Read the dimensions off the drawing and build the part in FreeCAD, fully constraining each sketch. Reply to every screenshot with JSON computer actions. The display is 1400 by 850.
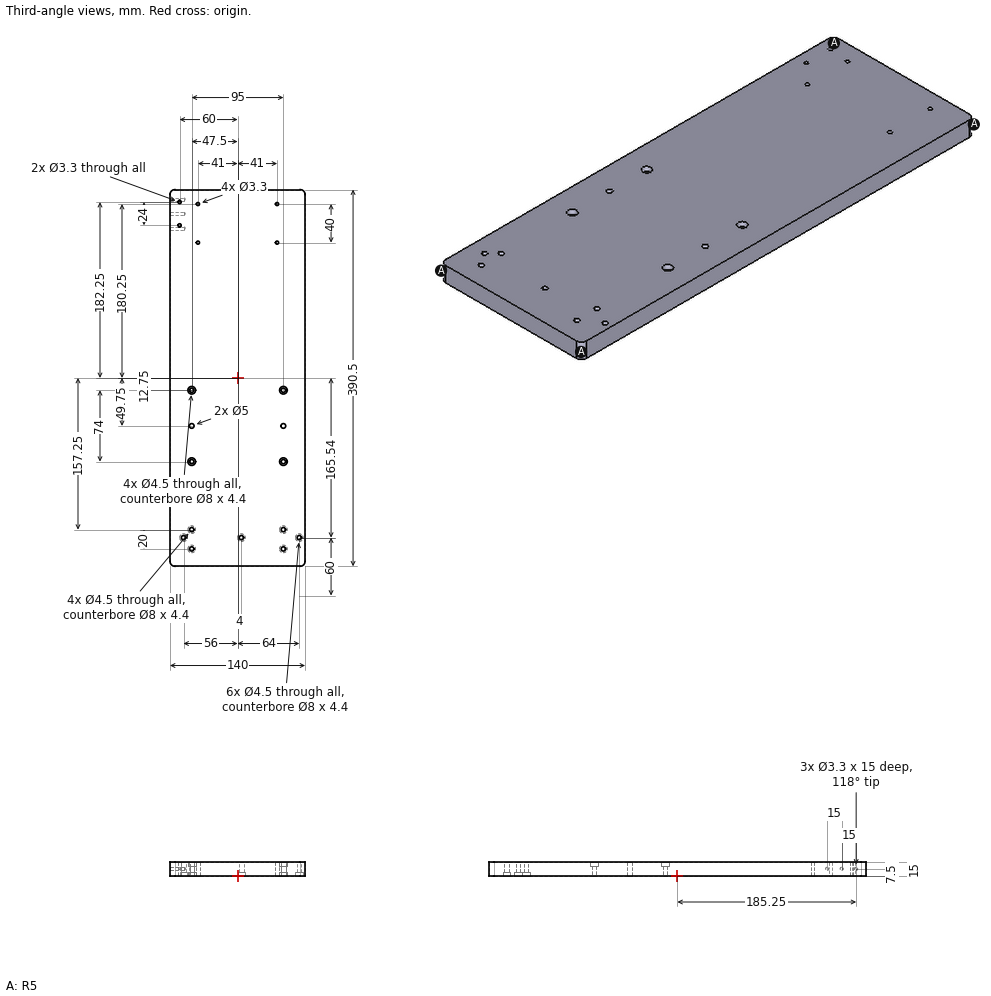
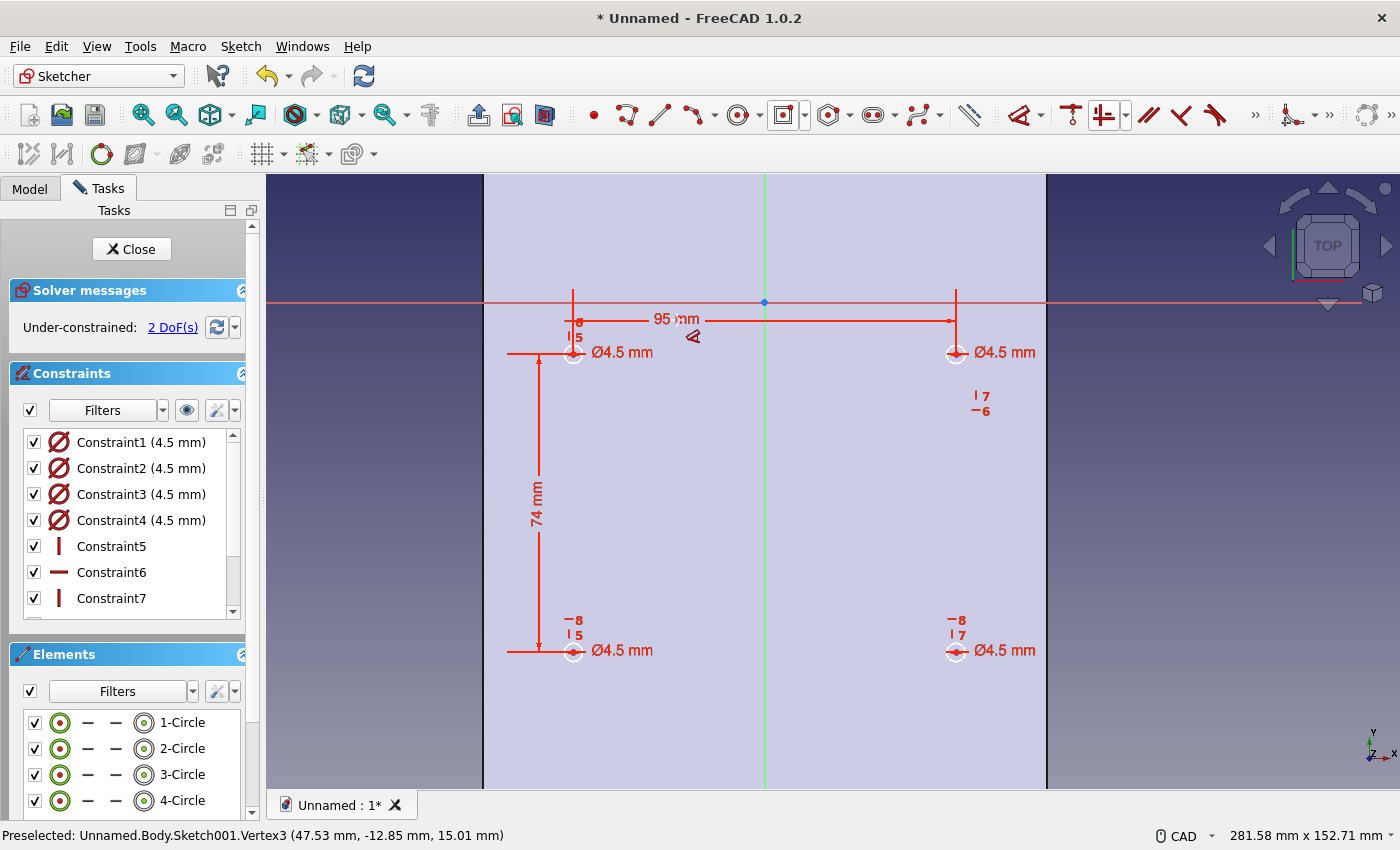
{"action": "left_click", "coordinate": [573, 354]}
{"action": "left_click", "coordinate": [669, 269]}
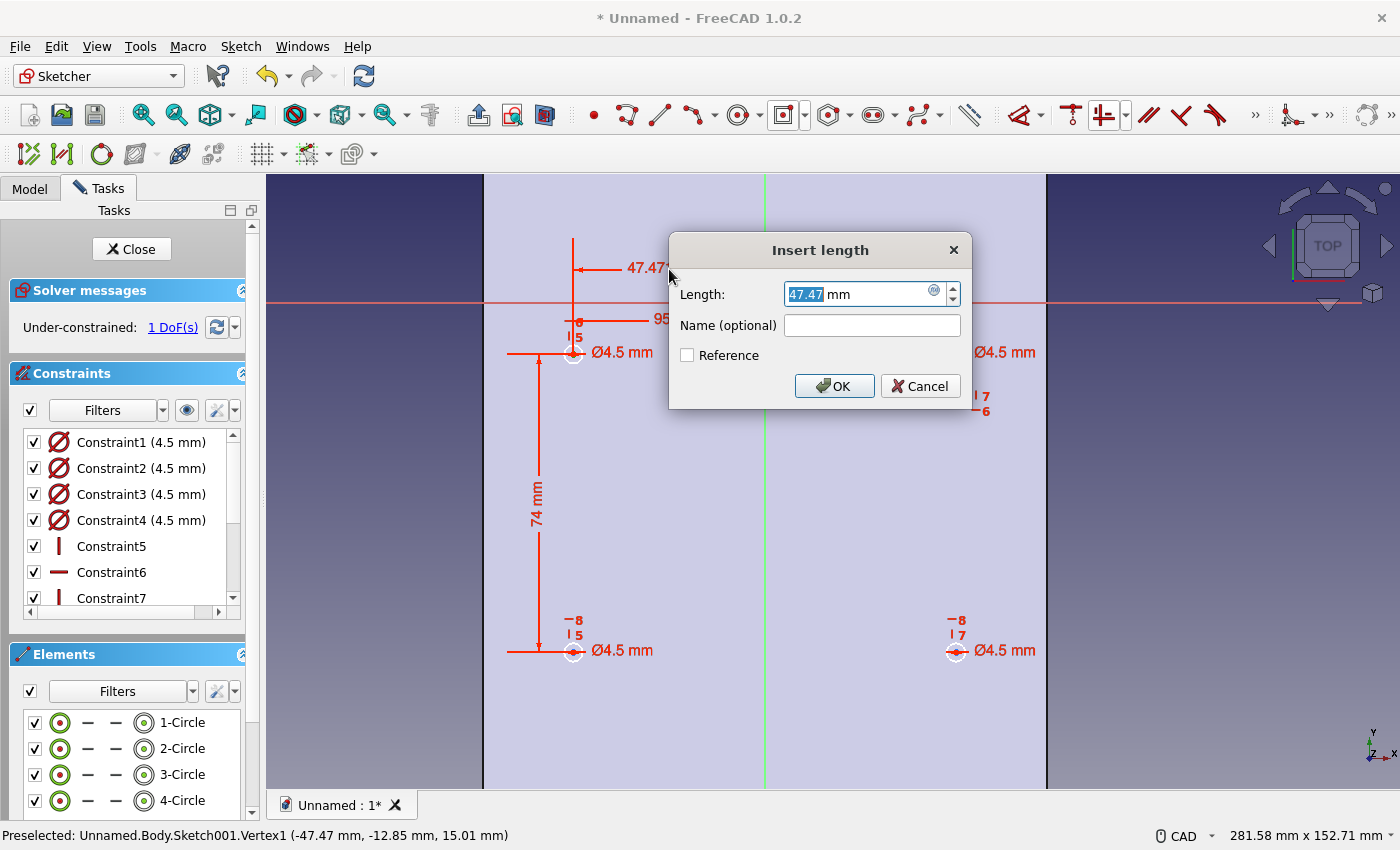
{"action": "type", "text": "47.5"}
{"action": "key", "text": "Return"}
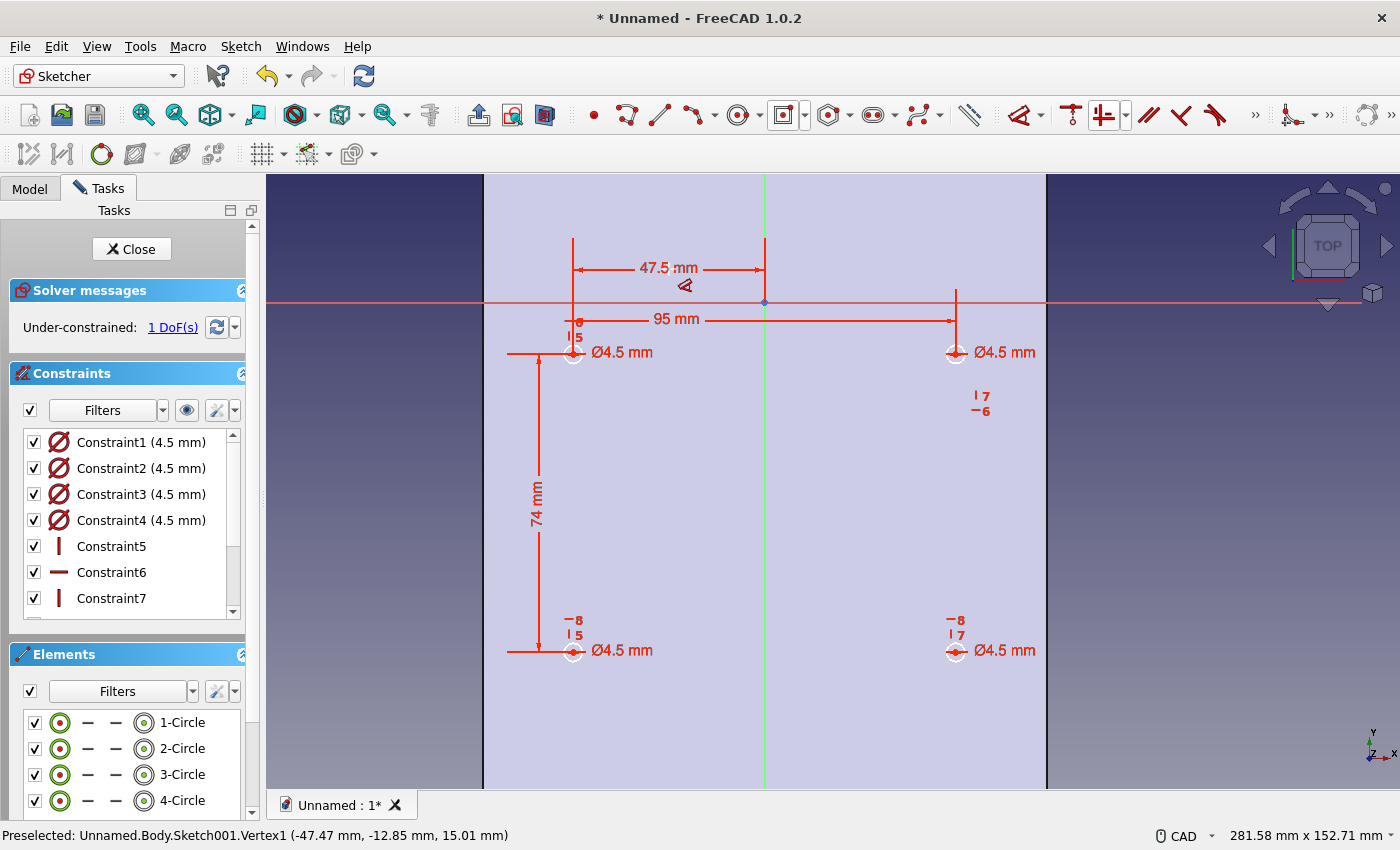
{"action": "left_click", "coordinate": [573, 354]}
{"action": "left_click", "coordinate": [539, 329]}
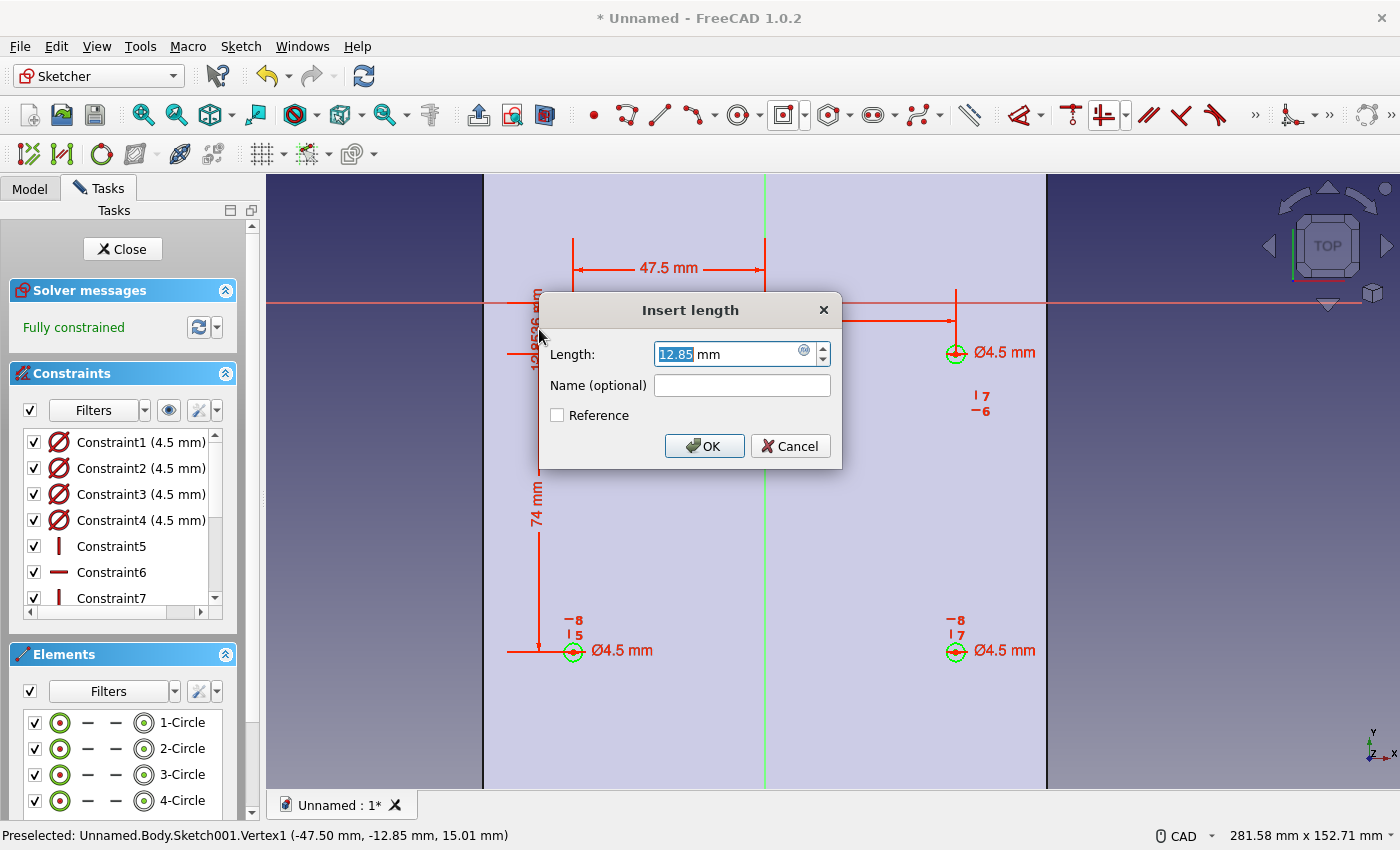
{"action": "type", "text": "12.75"}
{"action": "key", "text": "Return"}
{"action": "key", "text": "Escape"}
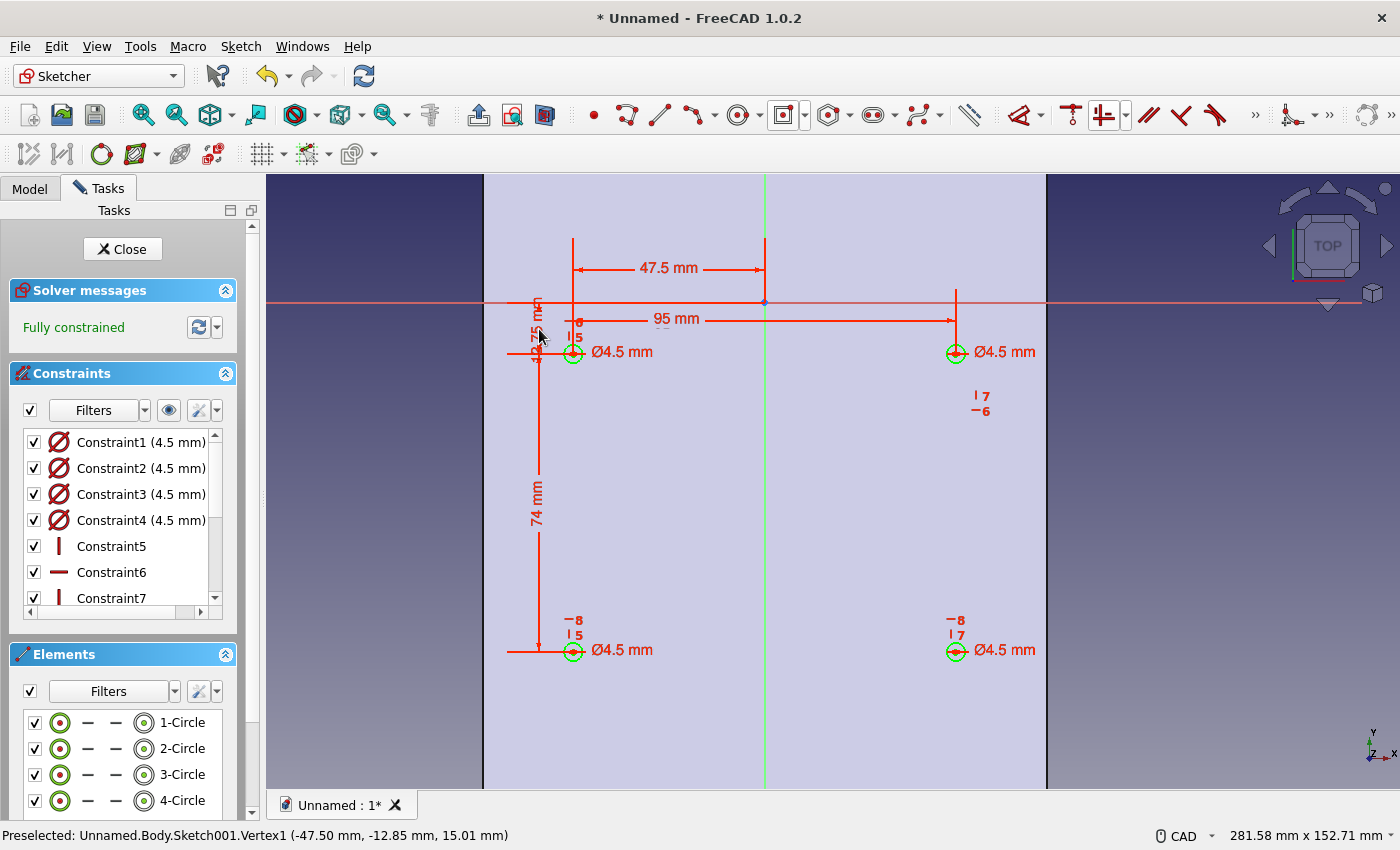
{"action": "left_click", "coordinate": [123, 249]}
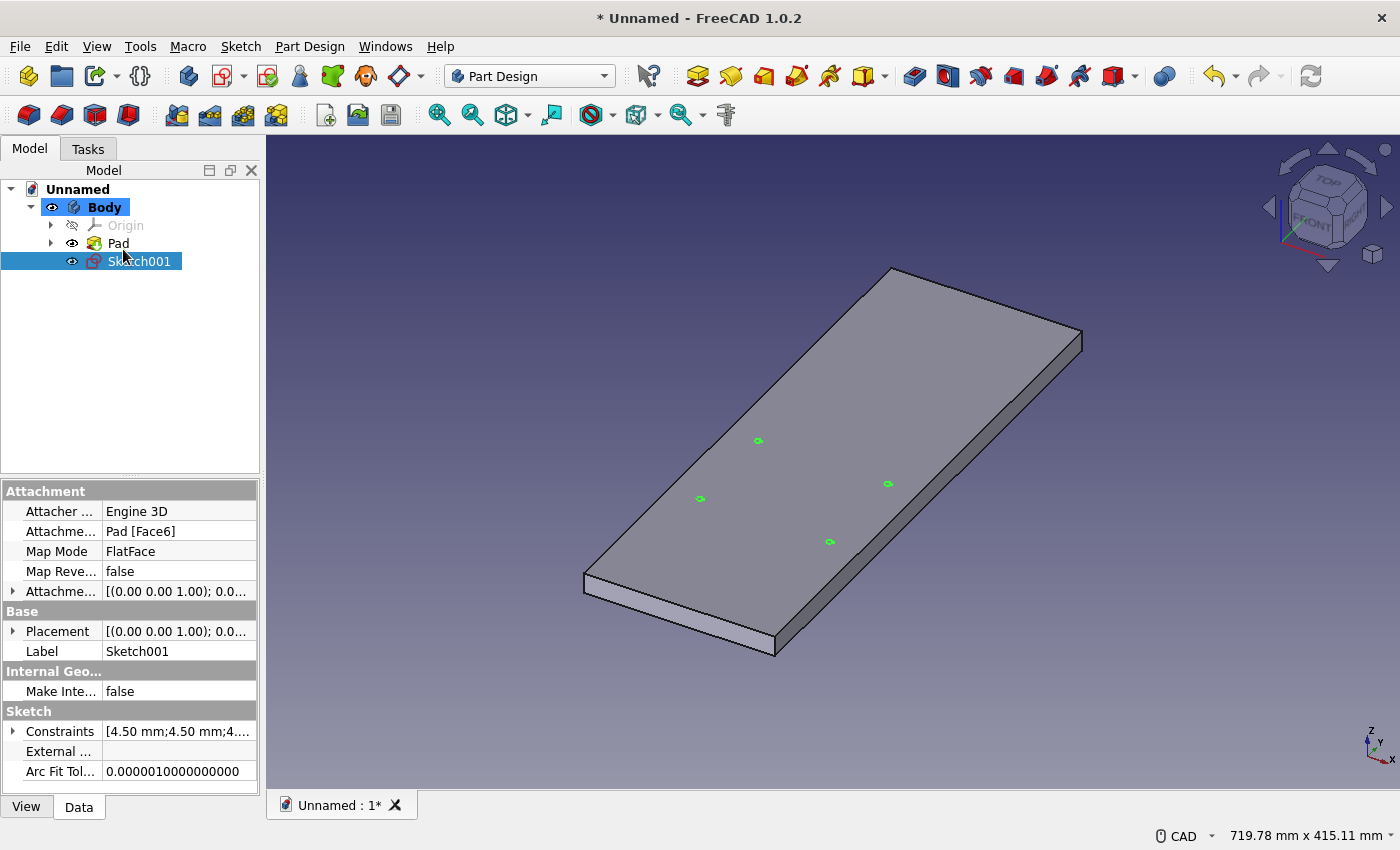
{"action": "left_click", "coordinate": [948, 76]}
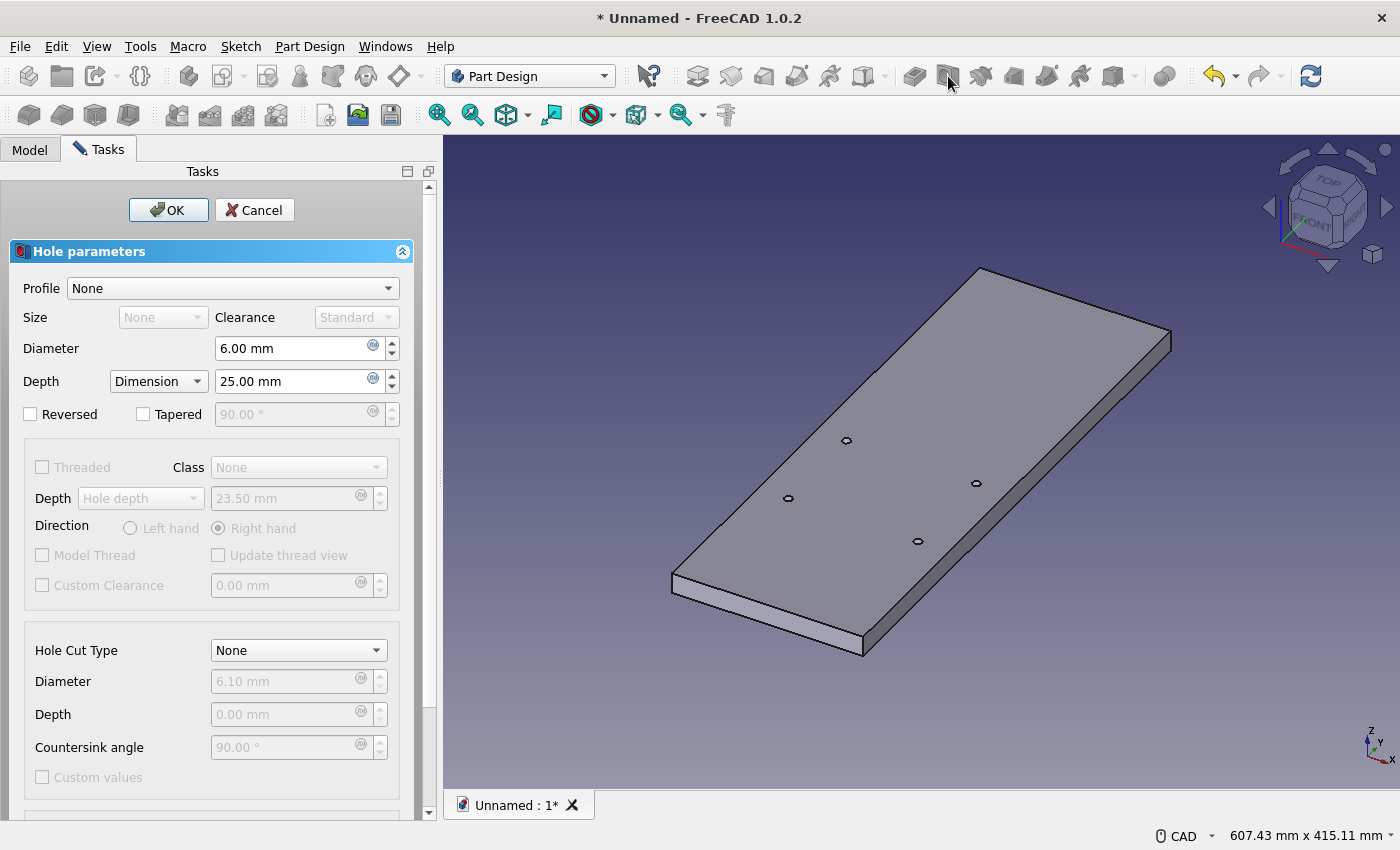
{"action": "triple_click", "coordinate": [300, 348]}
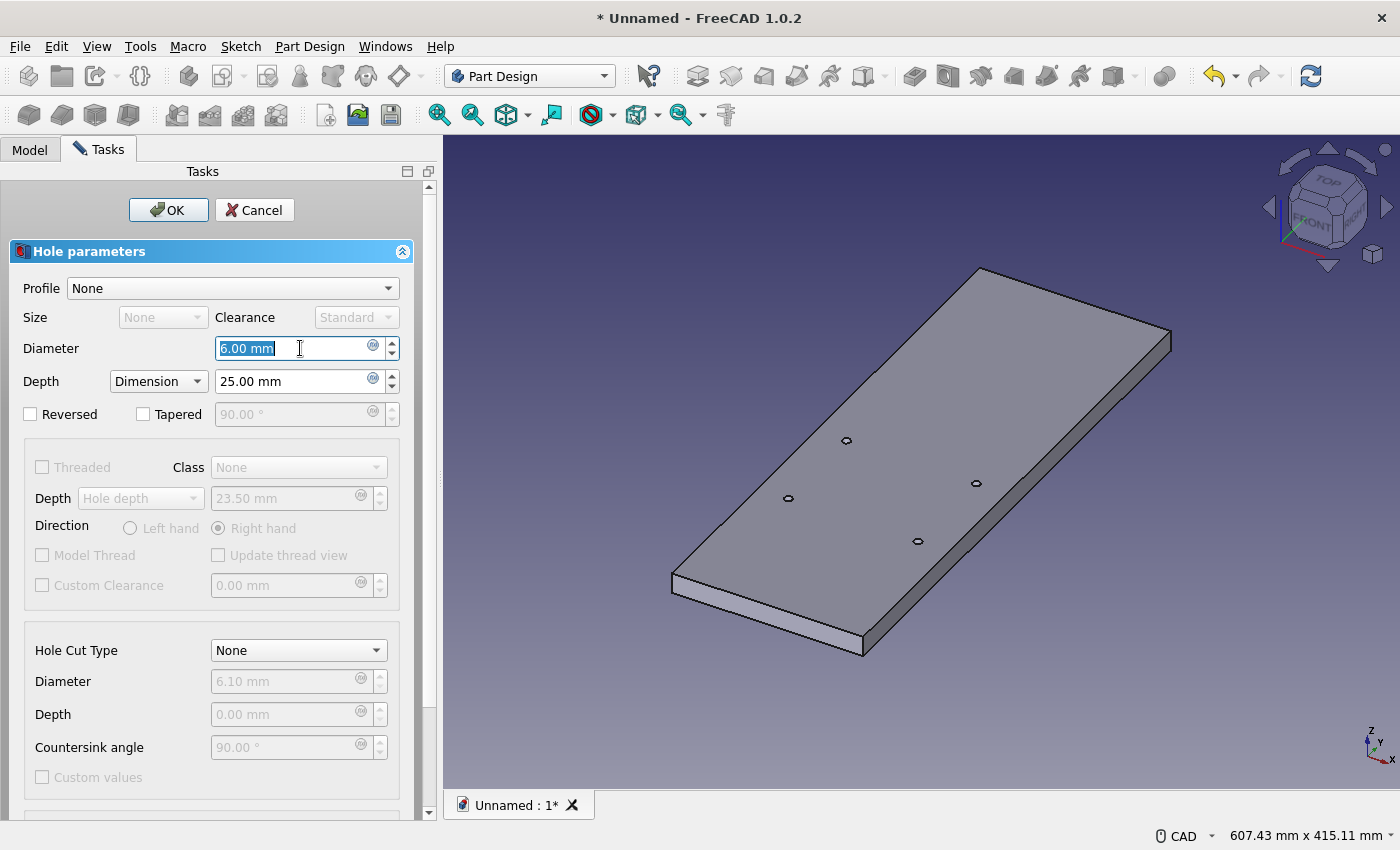
{"action": "type", "text": "4.5"}
{"action": "key", "text": "Tab"}